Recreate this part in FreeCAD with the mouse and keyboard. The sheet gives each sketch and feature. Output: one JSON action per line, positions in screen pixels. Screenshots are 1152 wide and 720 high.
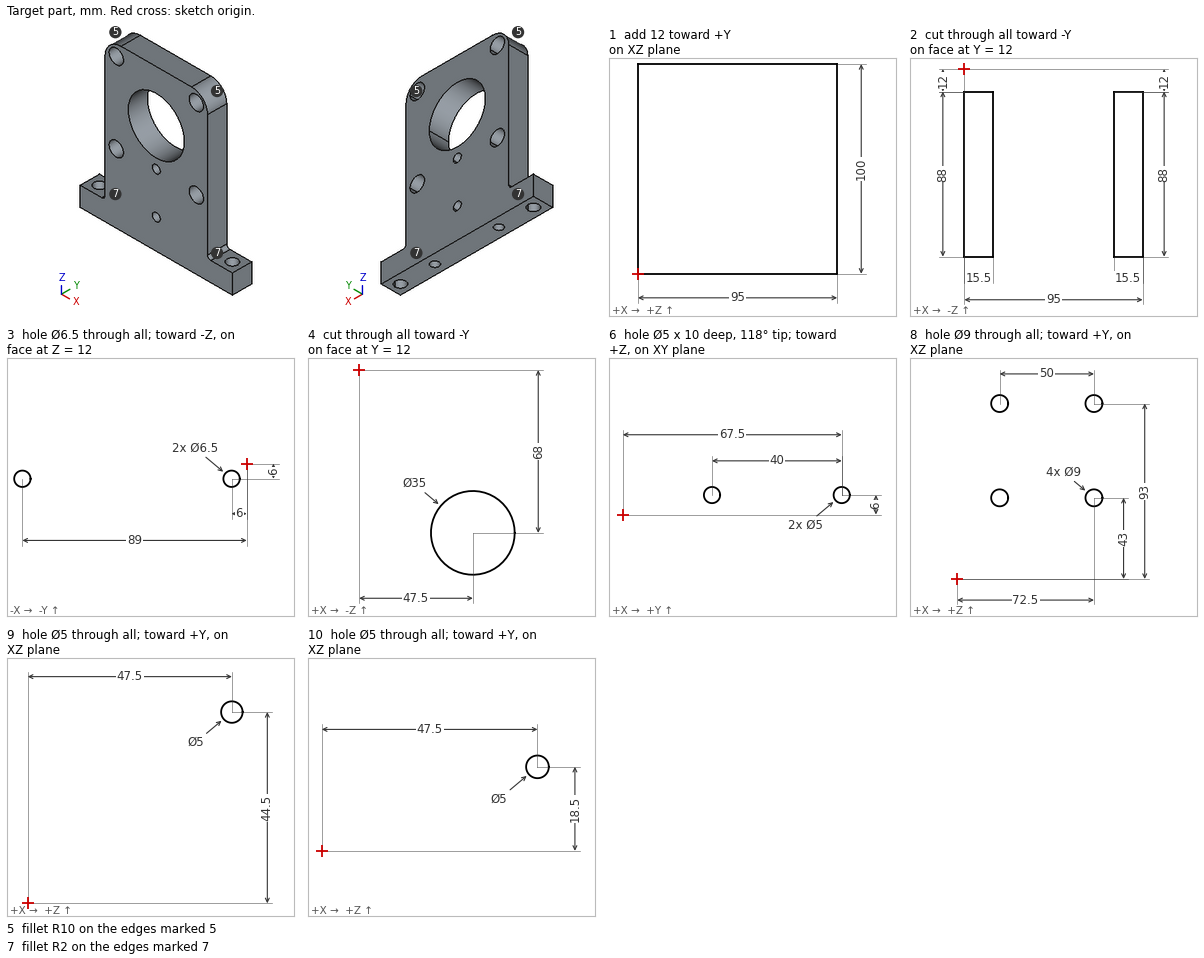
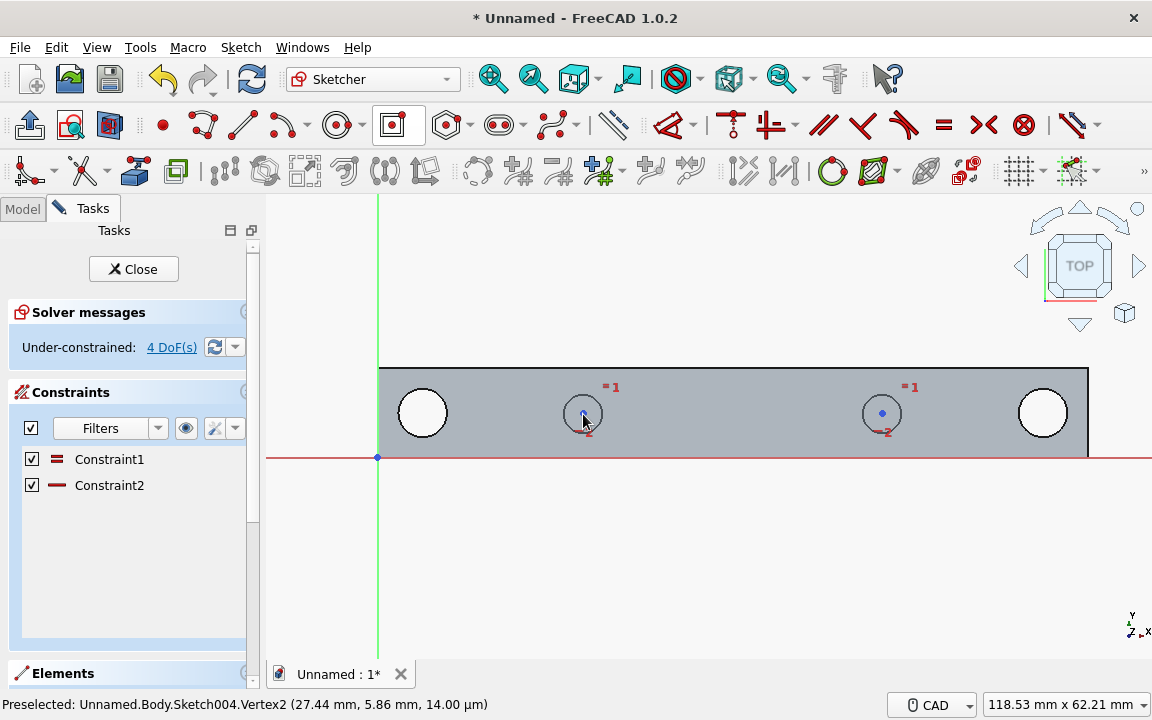
{"action": "left_click", "coordinate": [668, 126]}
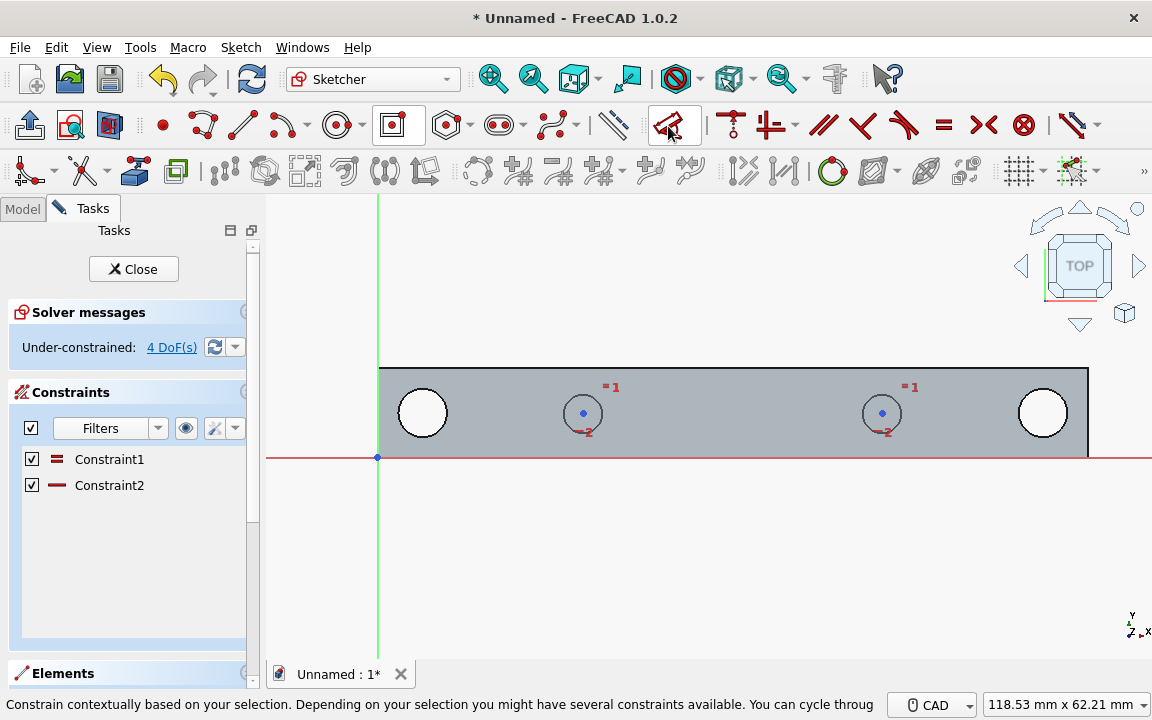
{"action": "left_click", "coordinate": [895, 400]}
{"action": "left_click", "coordinate": [917, 377]}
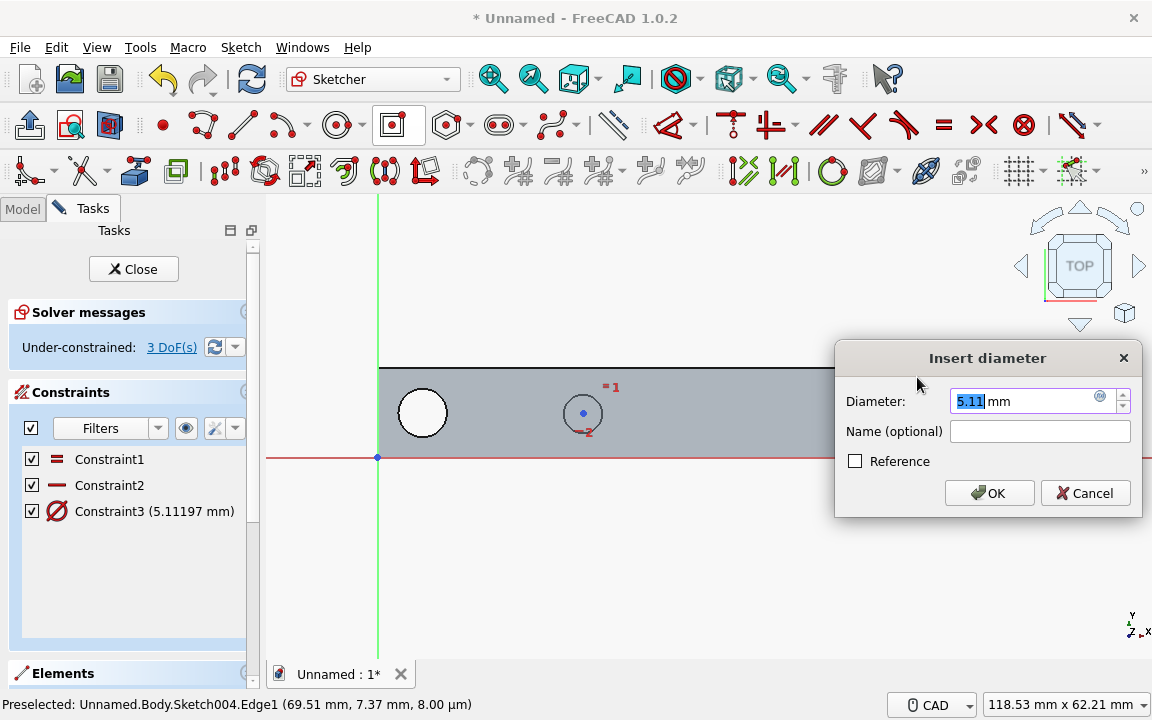
{"action": "type", "text": "5"}
{"action": "key", "text": "Return"}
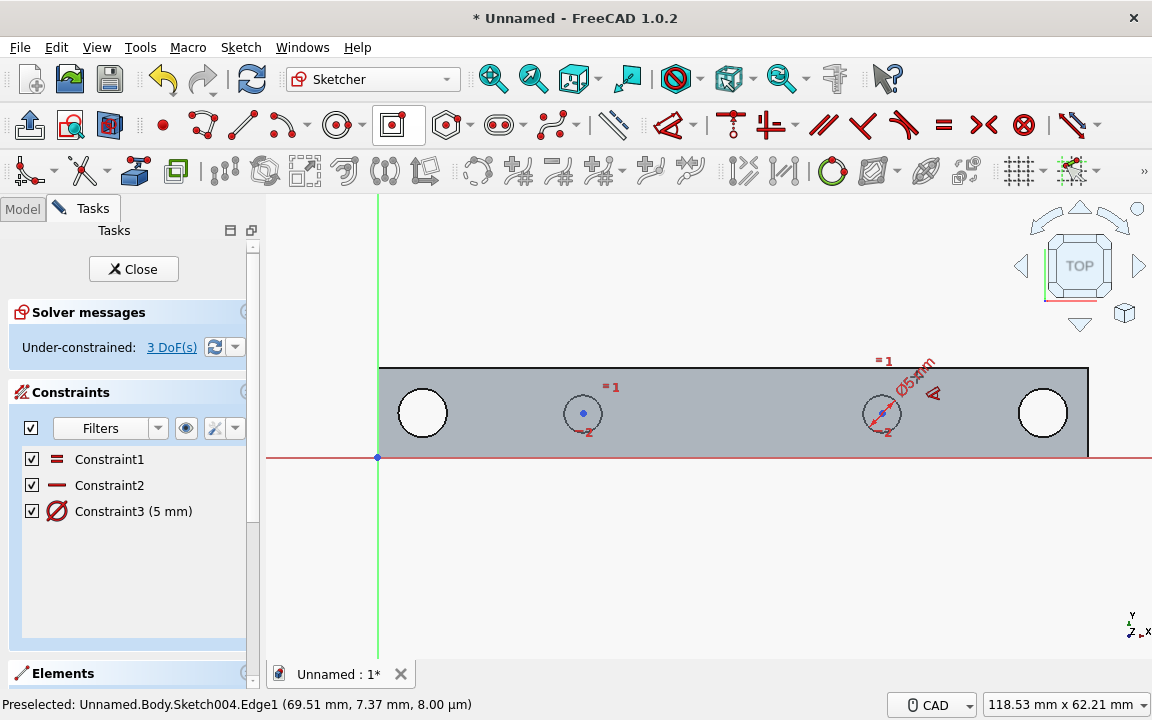
{"action": "left_click", "coordinate": [882, 414]}
{"action": "left_click", "coordinate": [344, 436]}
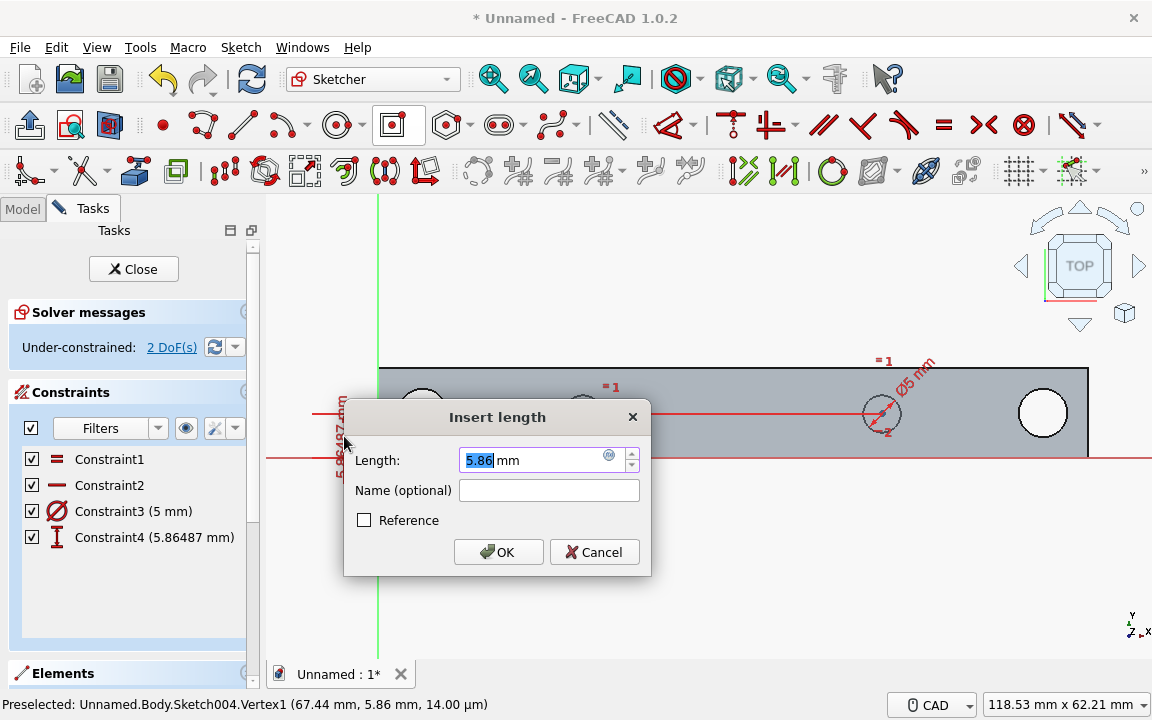
{"action": "type", "text": "6"}
{"action": "key", "text": "Return"}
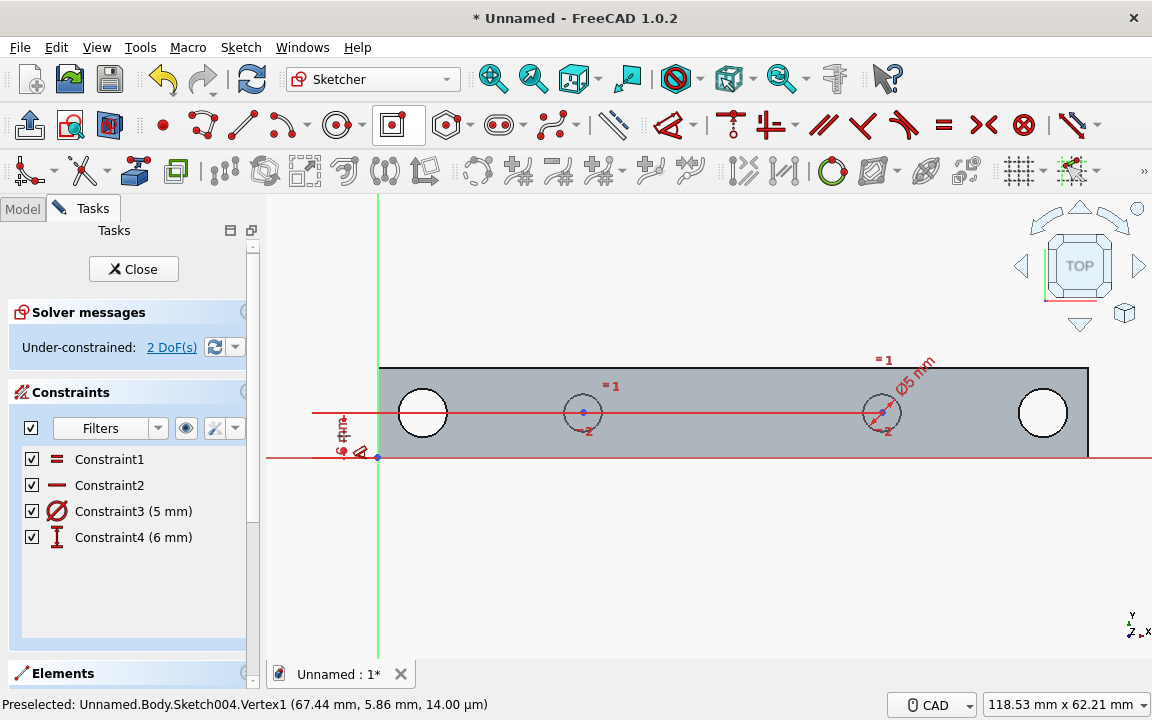
{"action": "left_click", "coordinate": [882, 413]}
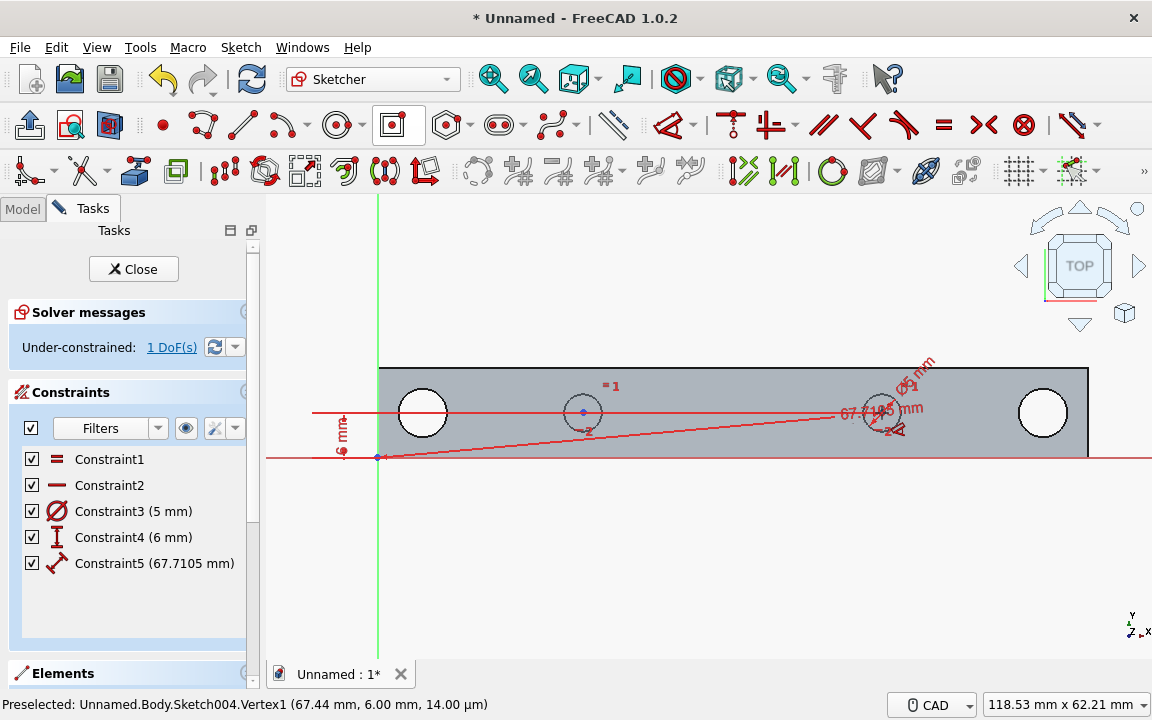
{"action": "left_click", "coordinate": [583, 413]}
{"action": "left_click", "coordinate": [732, 379]}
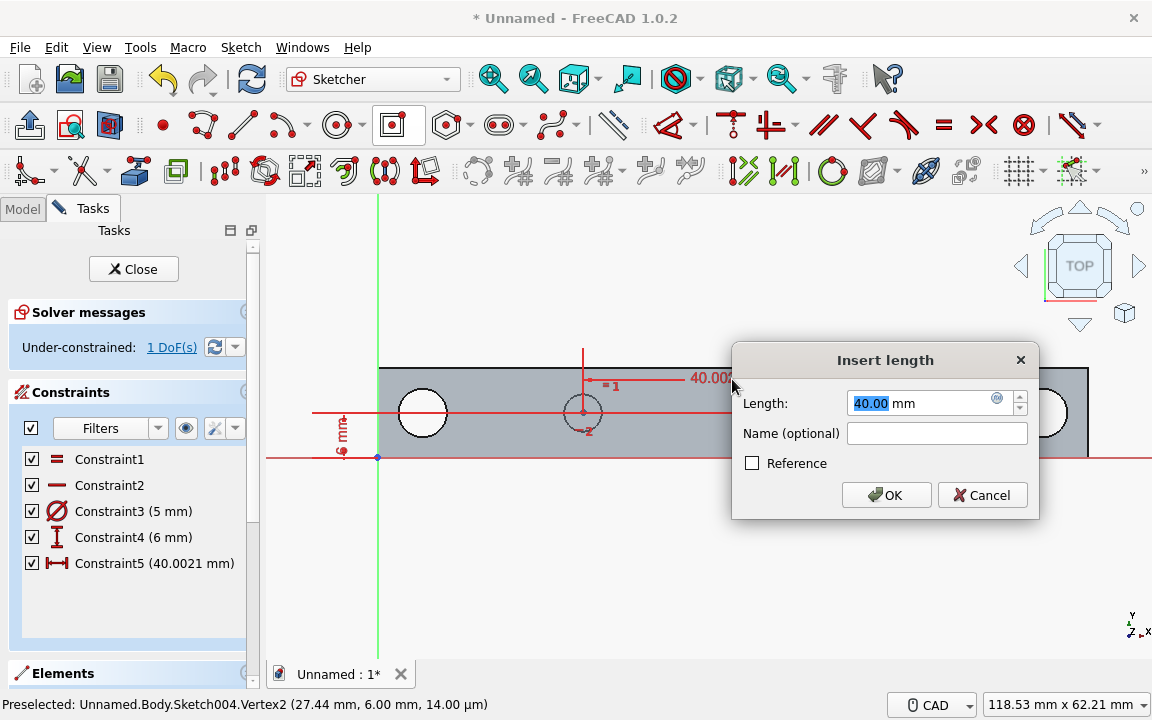
{"action": "type", "text": "40"}
{"action": "key", "text": "Return"}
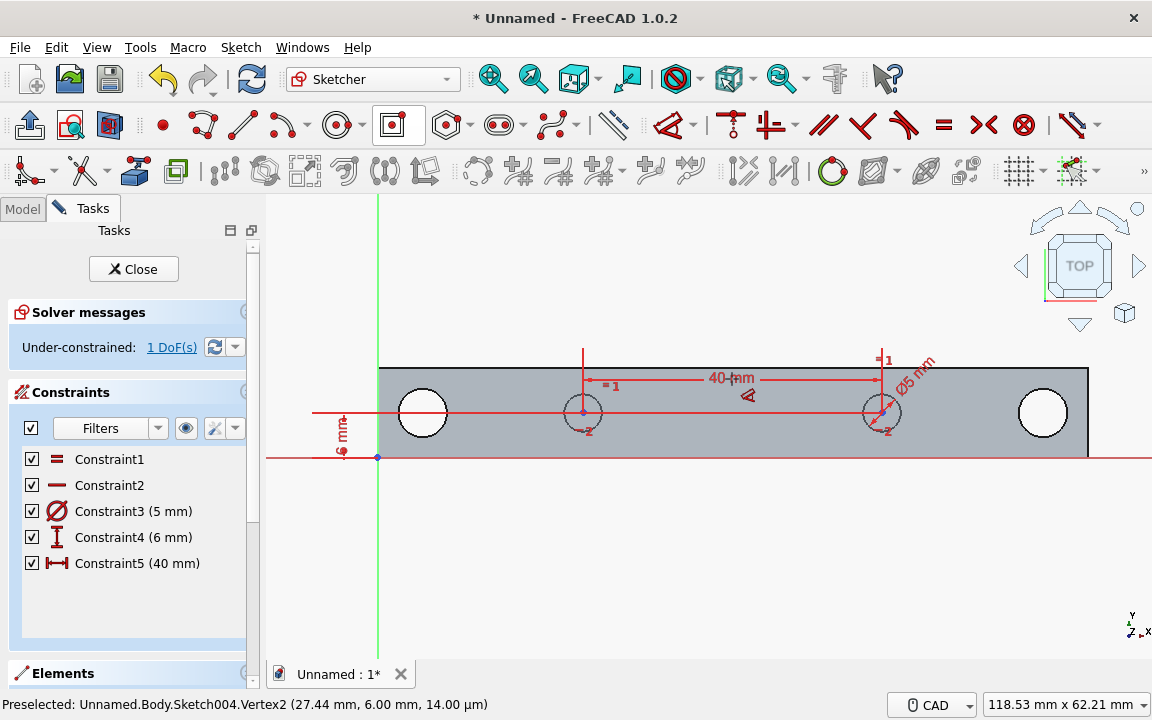
{"action": "left_click", "coordinate": [882, 413]}
{"action": "left_click", "coordinate": [630, 492]}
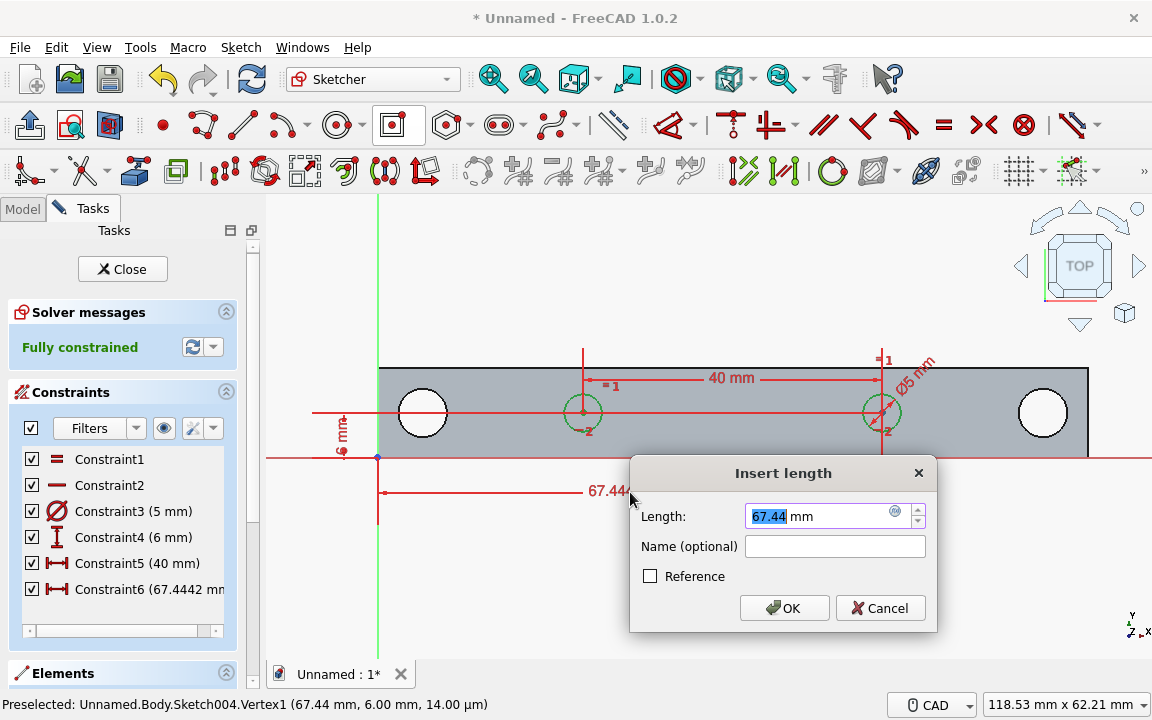
{"action": "type", "text": "67.5"}
{"action": "key", "text": "Return"}
{"action": "key", "text": "Escape"}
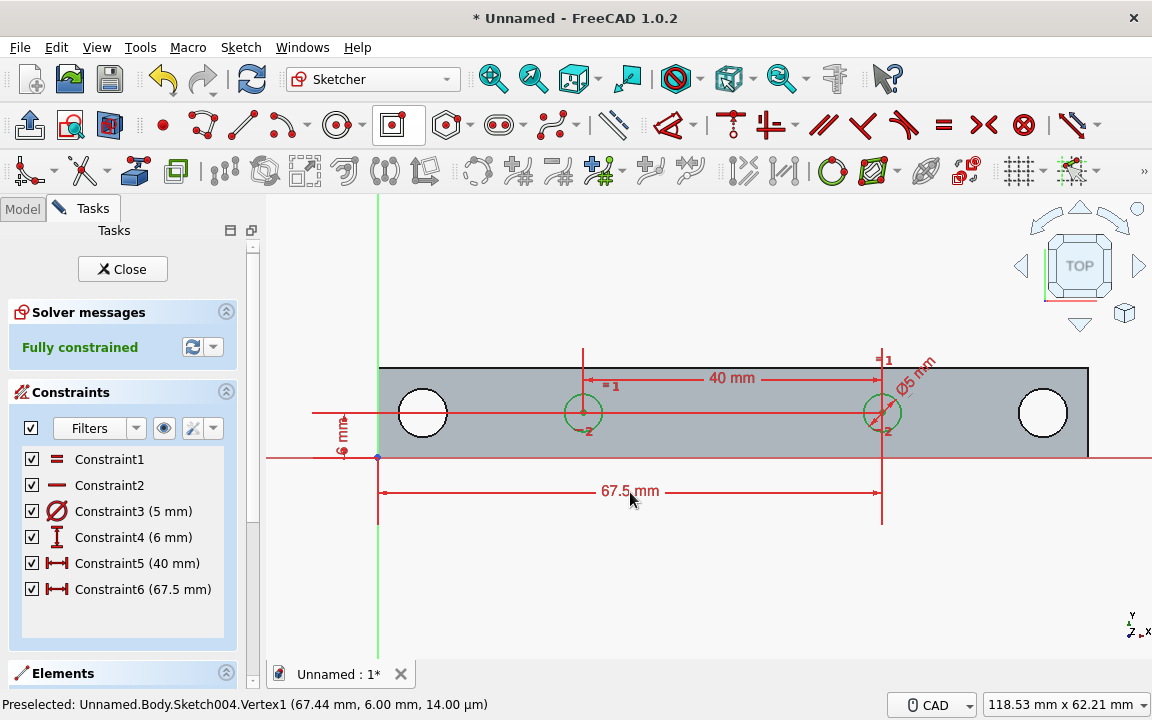
{"action": "left_click", "coordinate": [123, 269]}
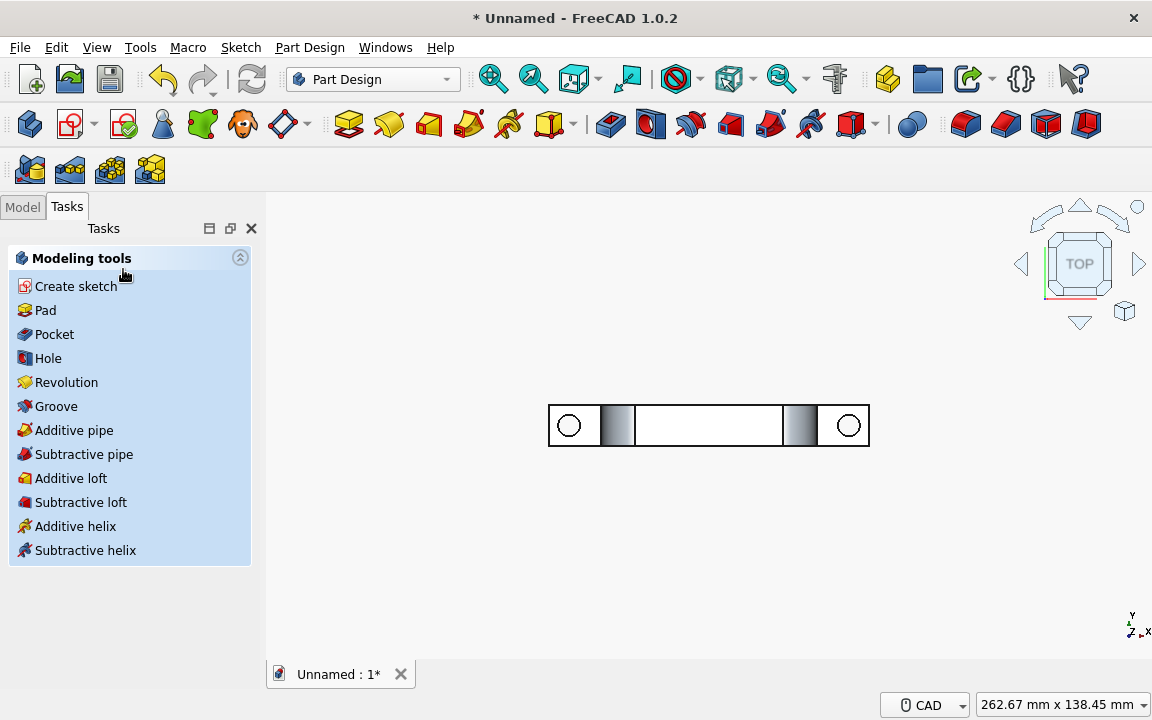
{"action": "left_click", "coordinate": [652, 124]}